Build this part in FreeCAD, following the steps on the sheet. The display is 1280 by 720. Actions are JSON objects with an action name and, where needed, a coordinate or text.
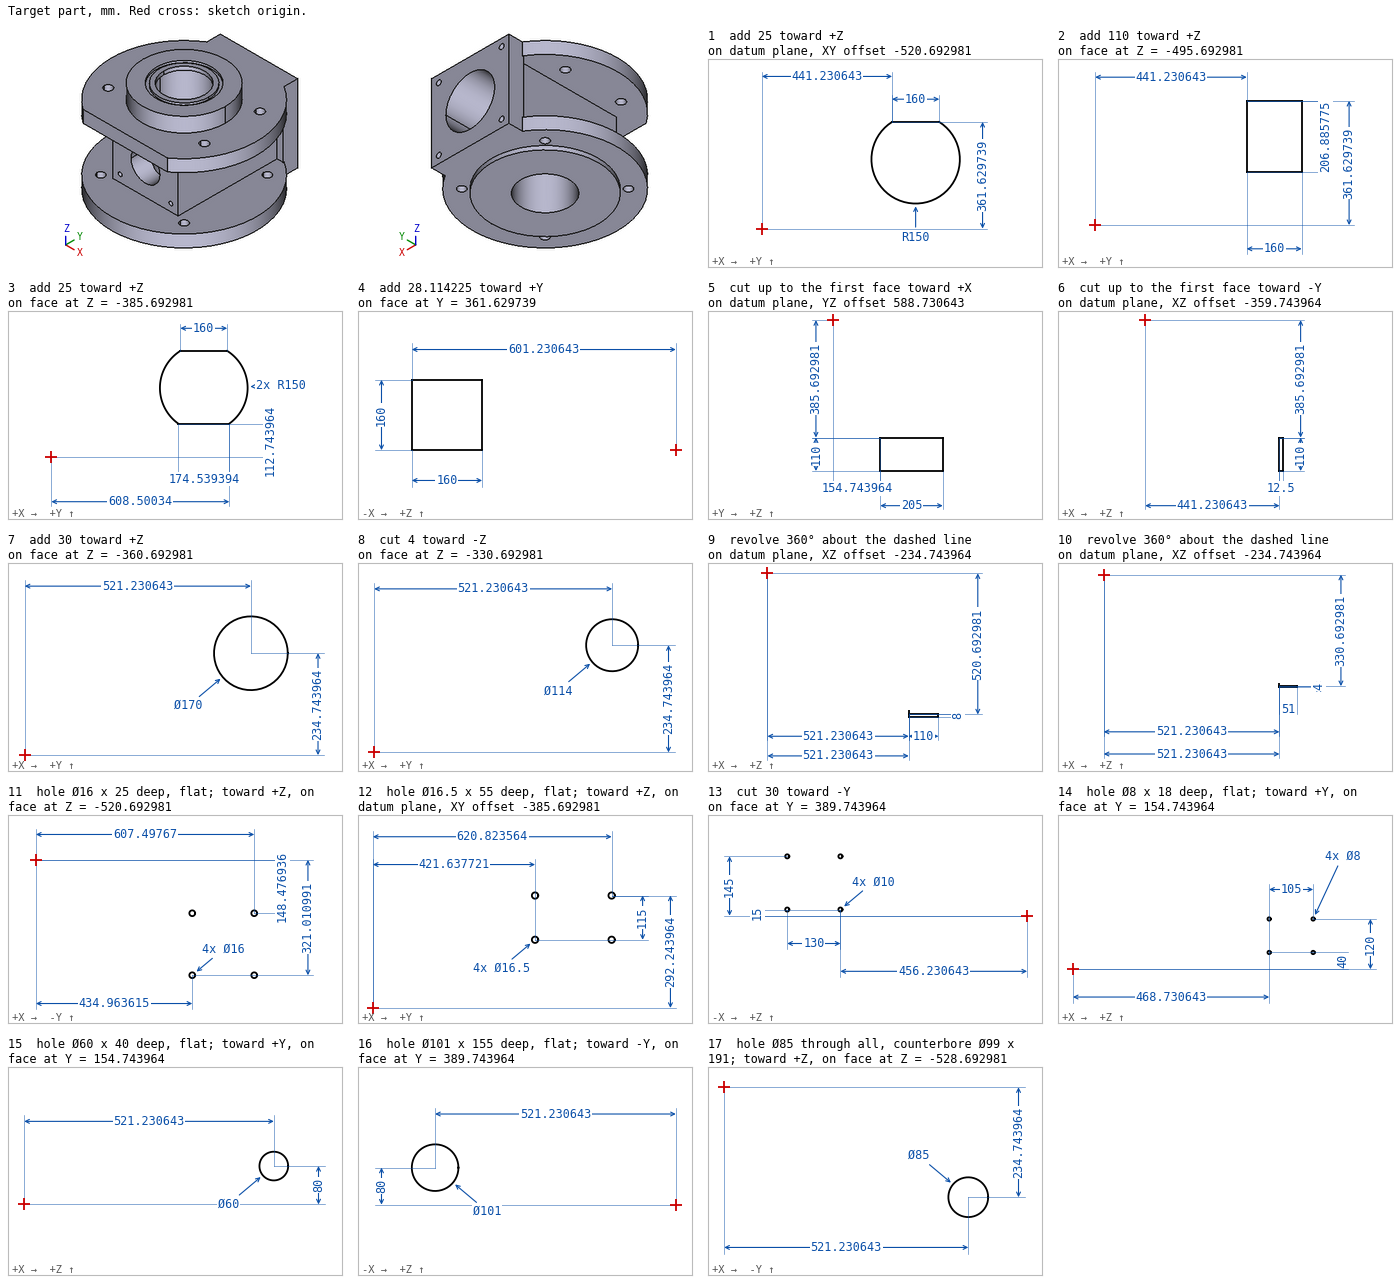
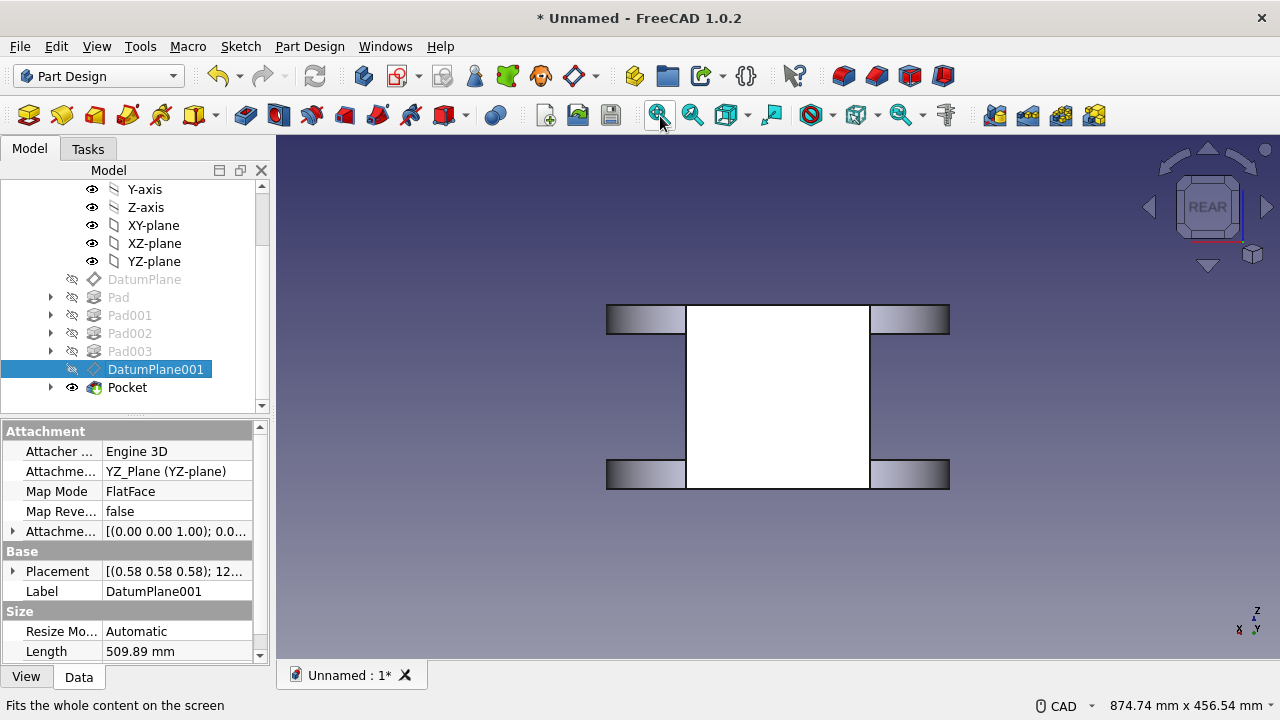
{"action": "key", "text": "0"}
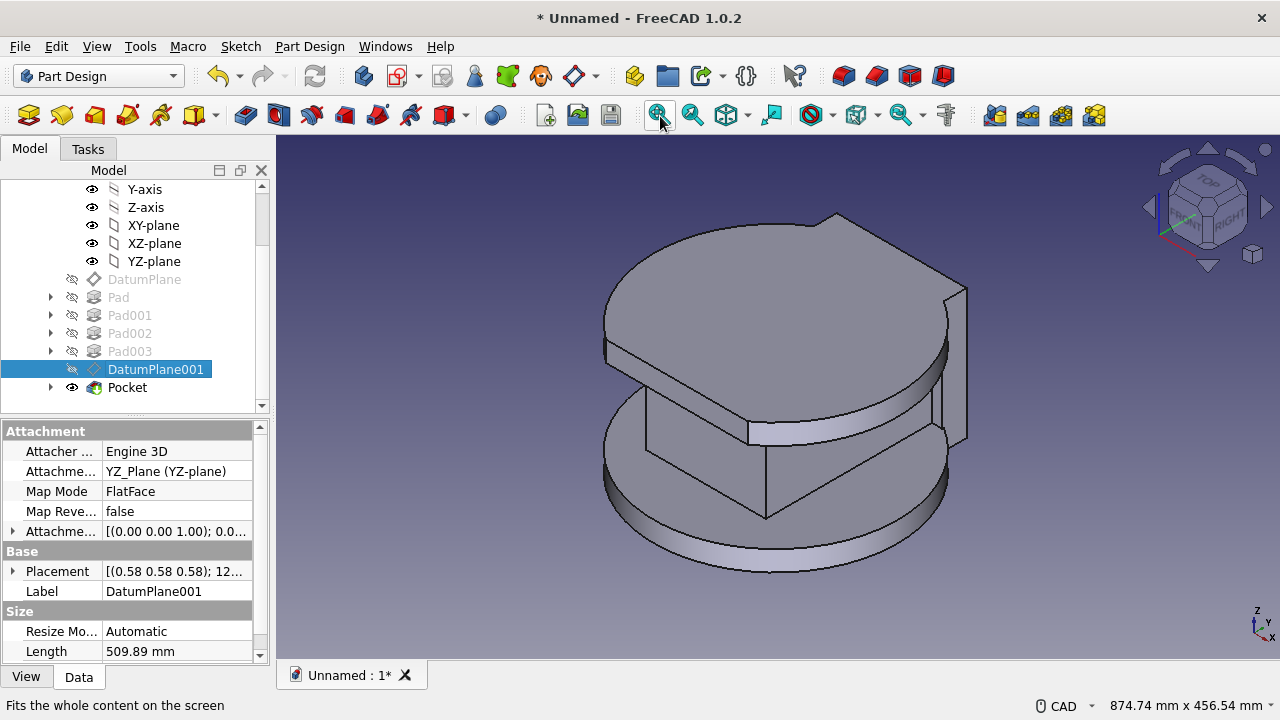
{"action": "key", "text": "1"}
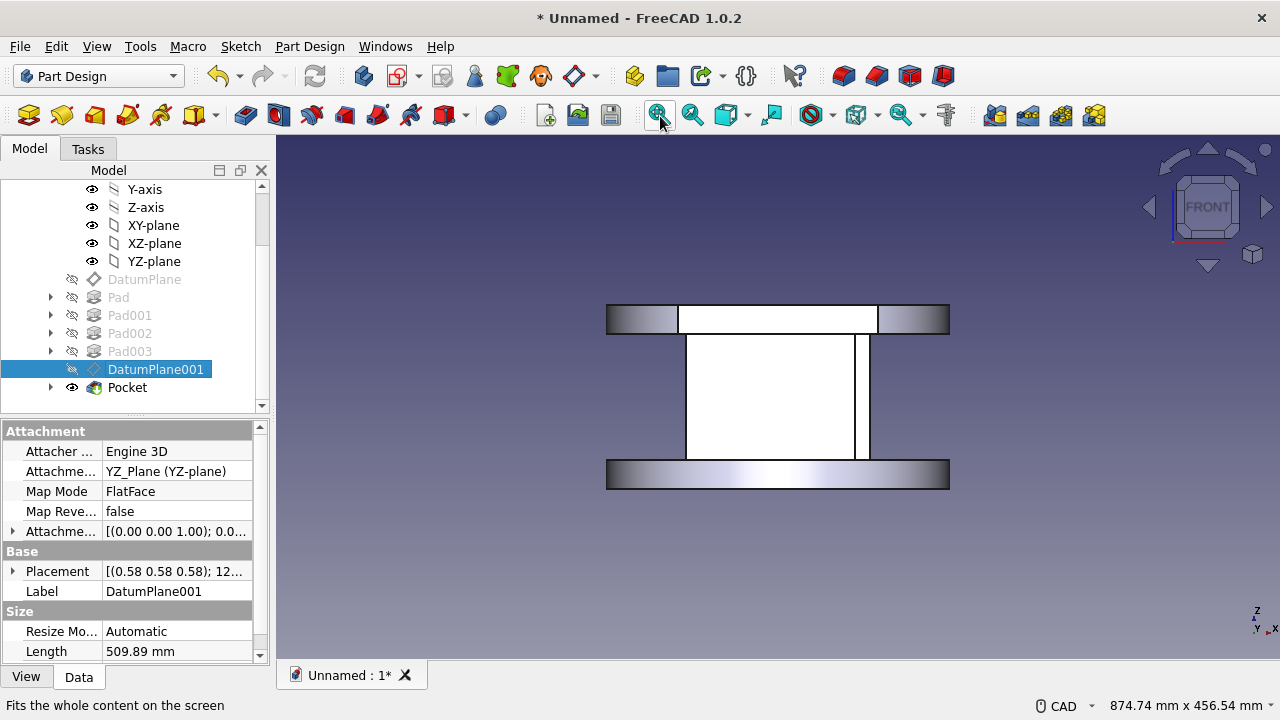
{"action": "left_click", "coordinate": [660, 116]}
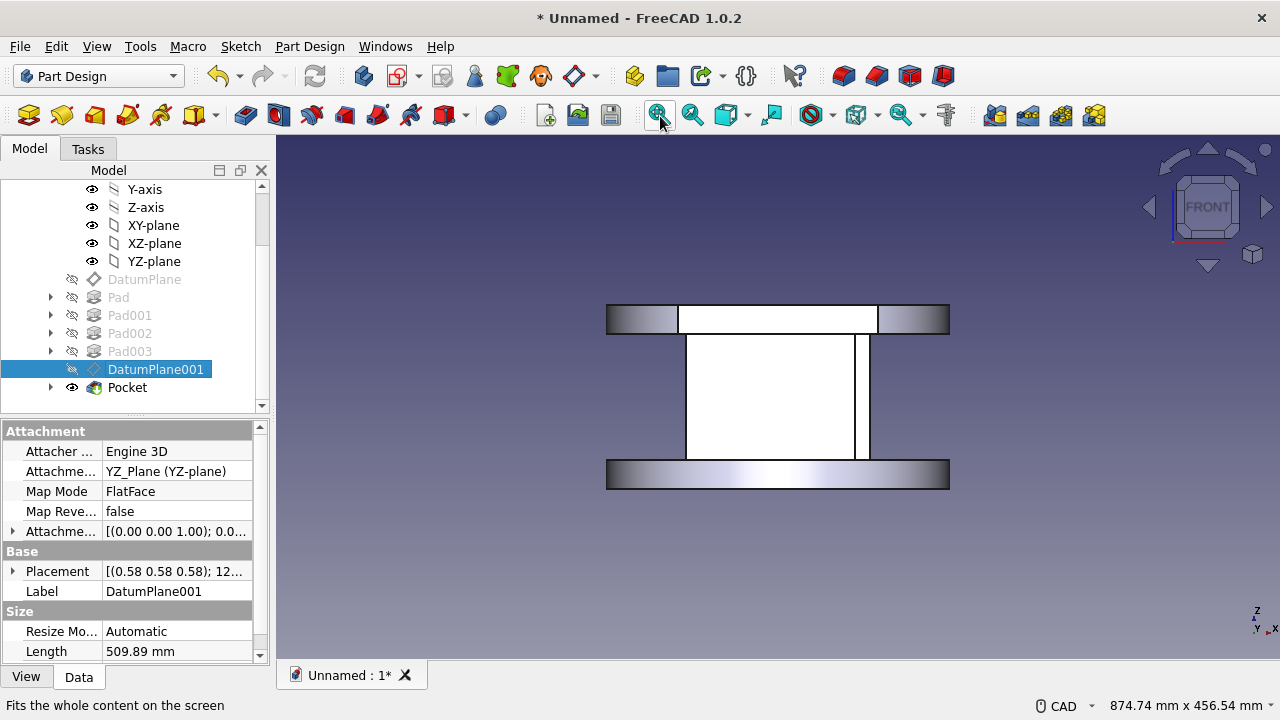
{"action": "key", "text": "2"}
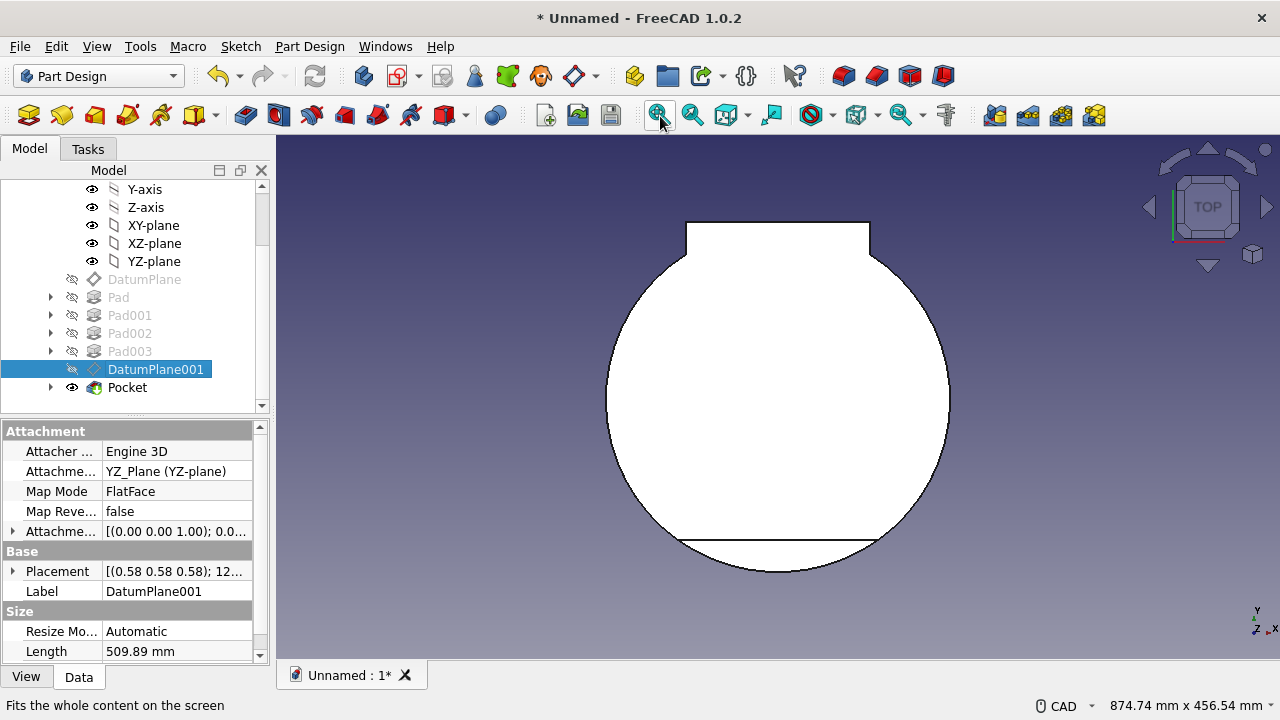
{"action": "scroll", "coordinate": [161, 293], "scroll_direction": "down", "scroll_amount": 3}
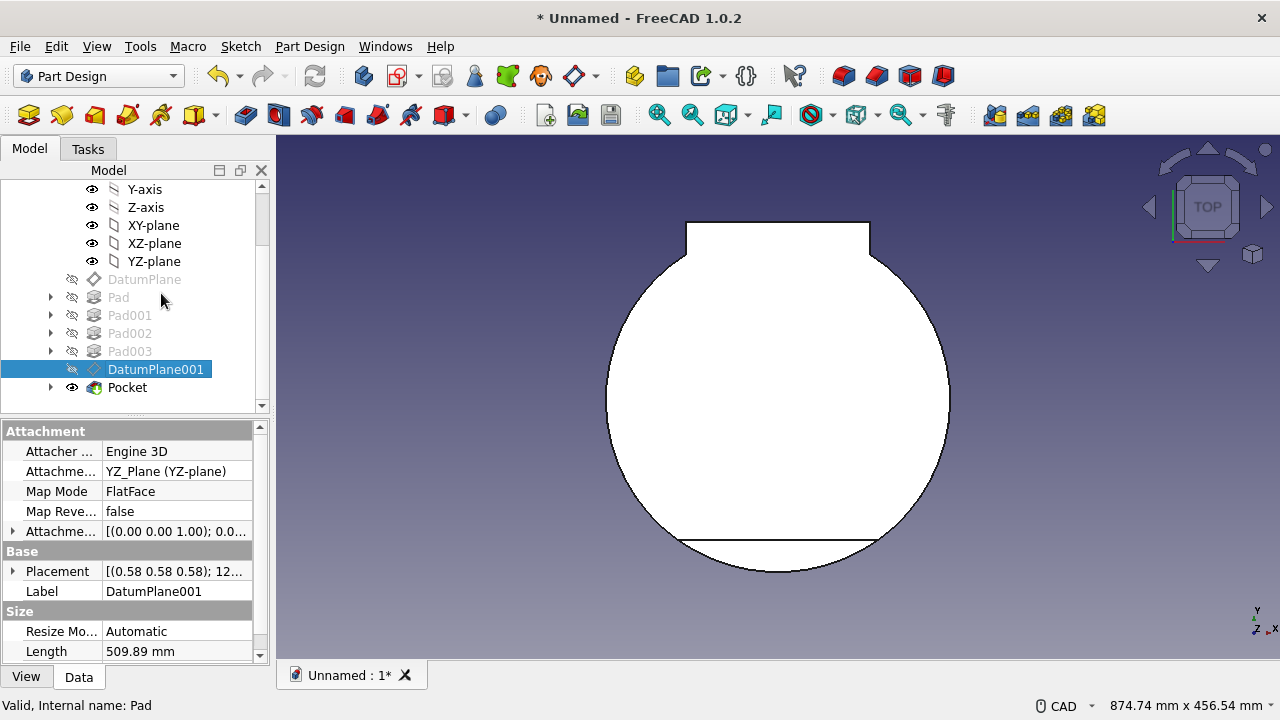
{"action": "scroll", "coordinate": [161, 293], "scroll_direction": "up", "scroll_amount": 15}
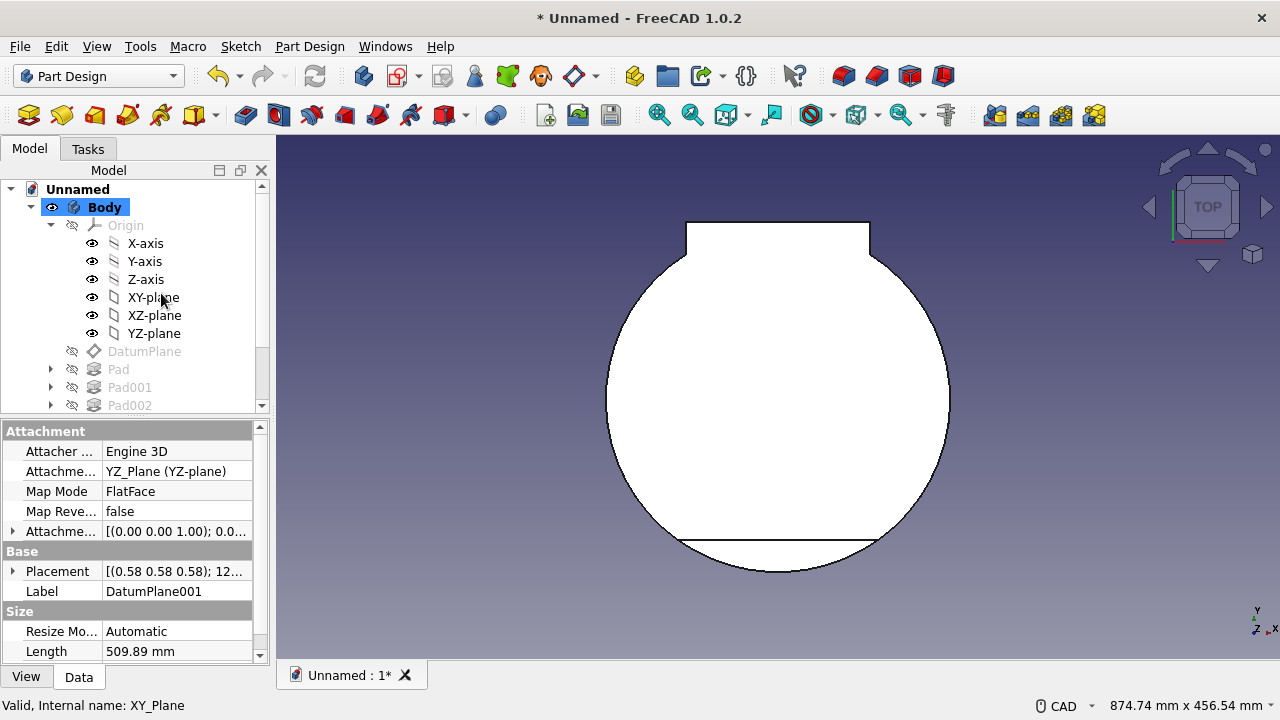
{"action": "left_click", "coordinate": [137, 315]}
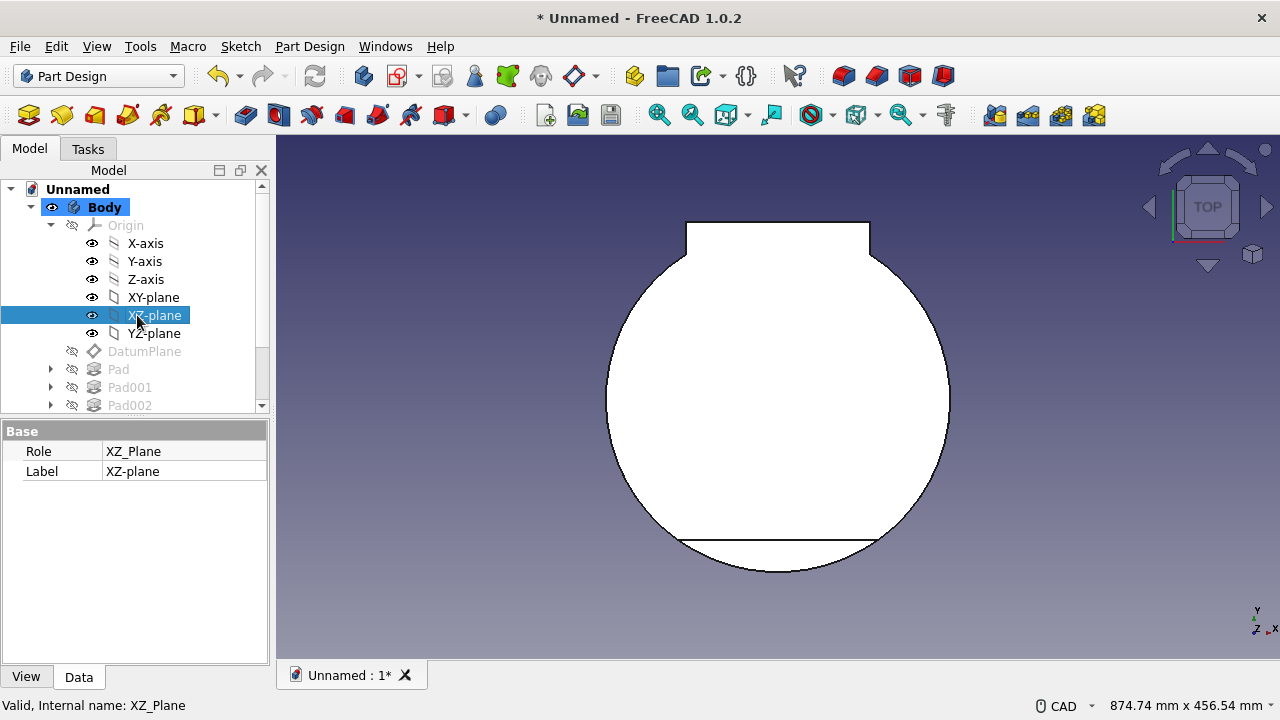
{"action": "left_click", "coordinate": [574, 76]}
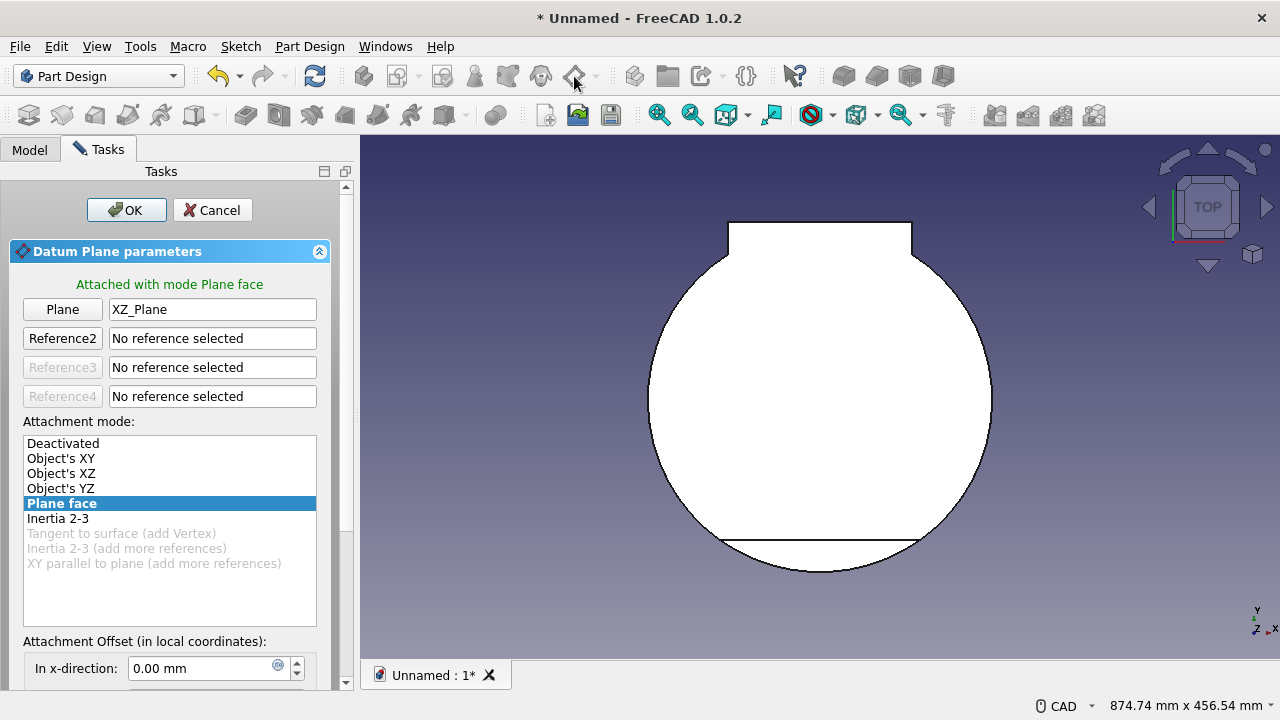
{"action": "scroll", "coordinate": [346, 436], "scroll_direction": "down", "scroll_amount": 2}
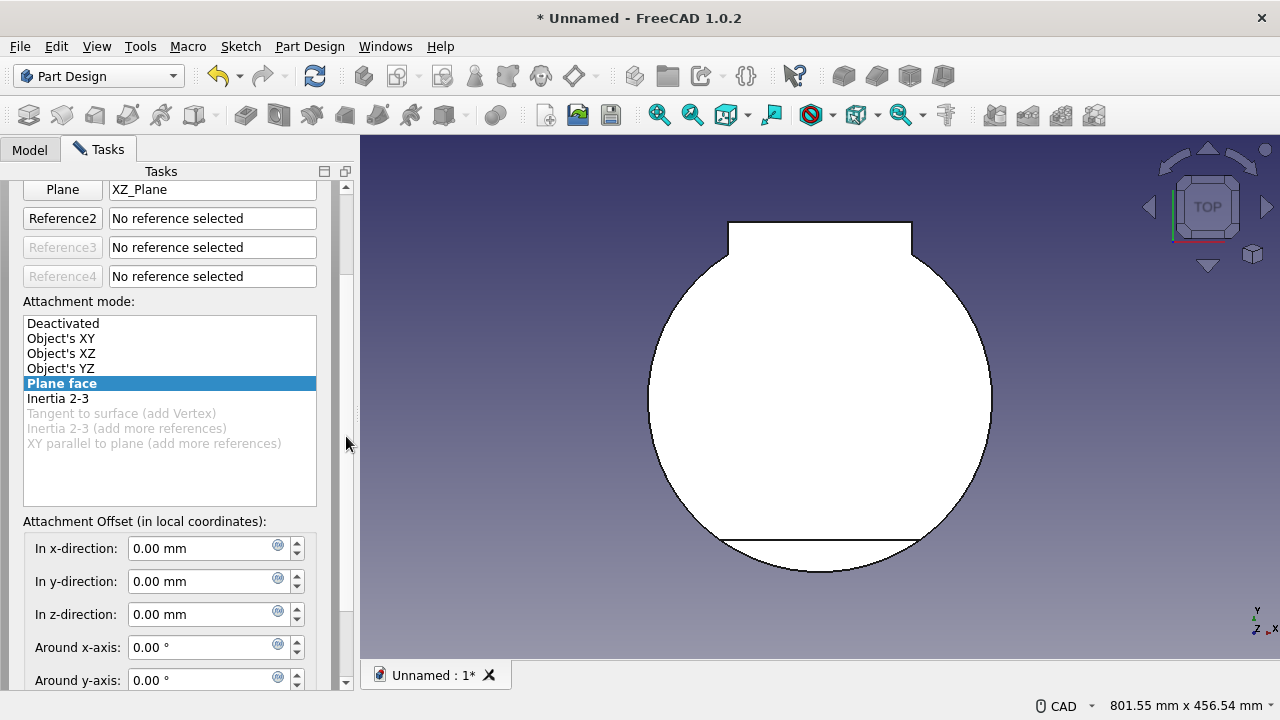
{"action": "triple_click", "coordinate": [210, 614]}